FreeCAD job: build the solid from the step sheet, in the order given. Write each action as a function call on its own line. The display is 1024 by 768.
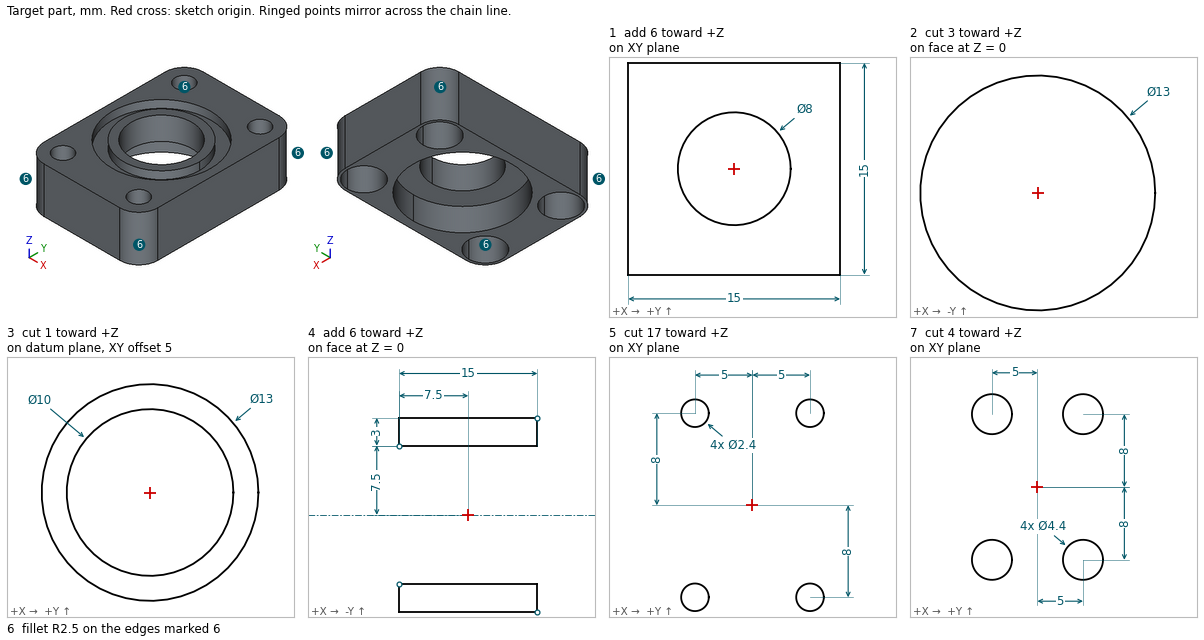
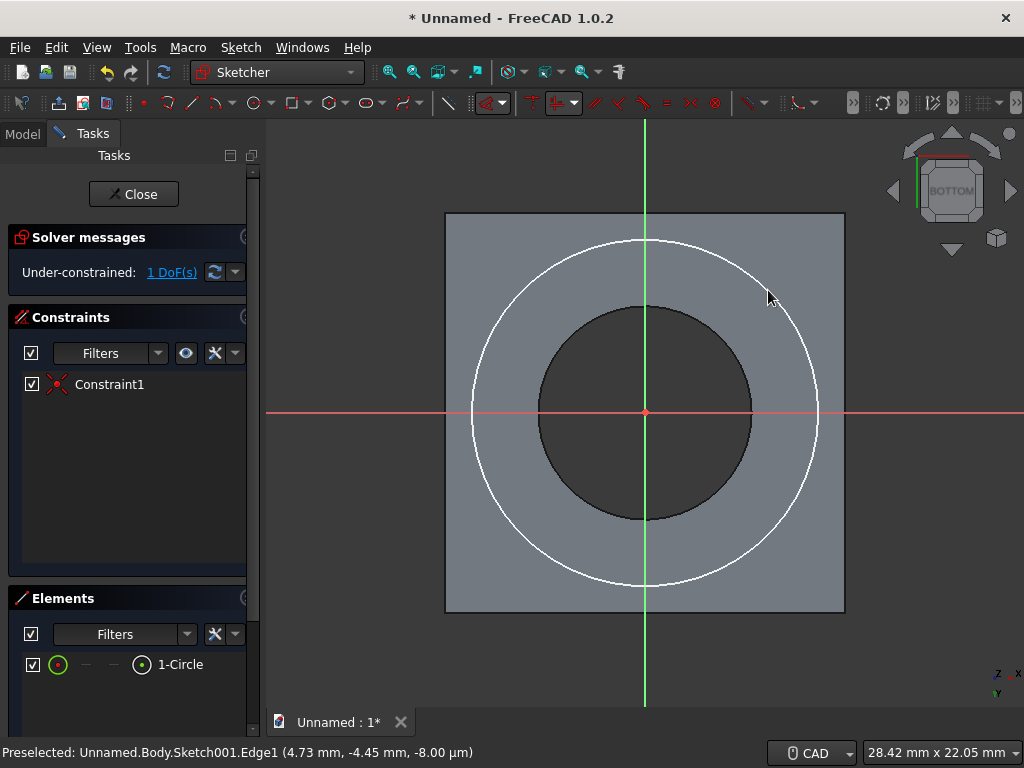
click(486, 104)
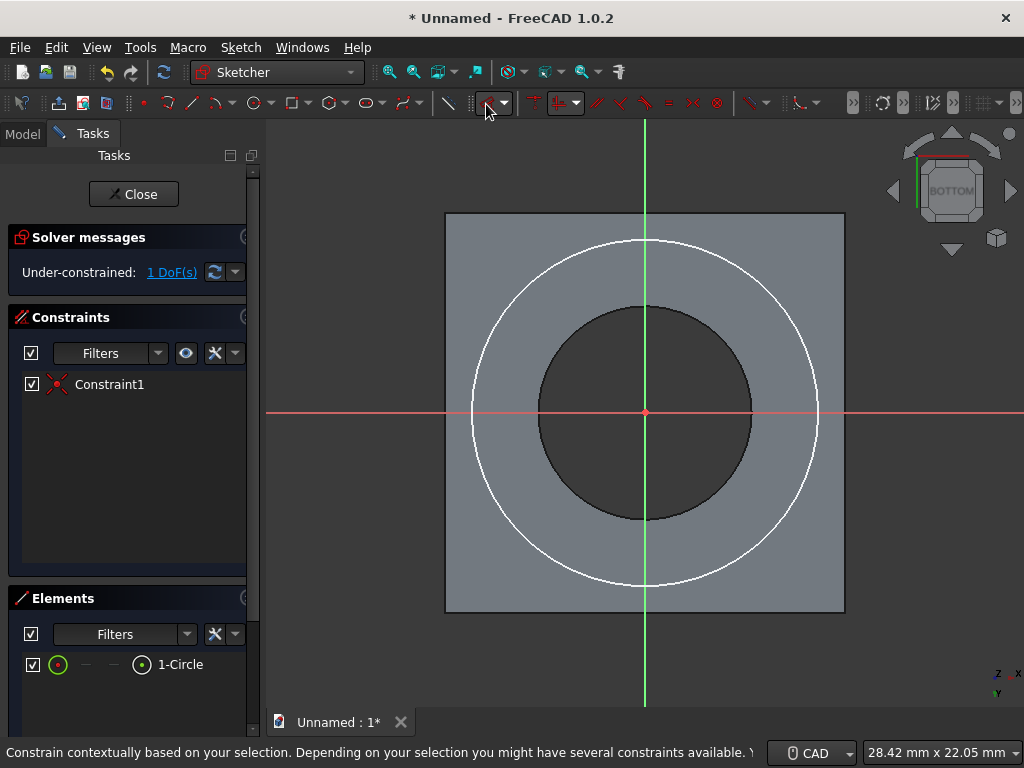
click(767, 290)
click(790, 267)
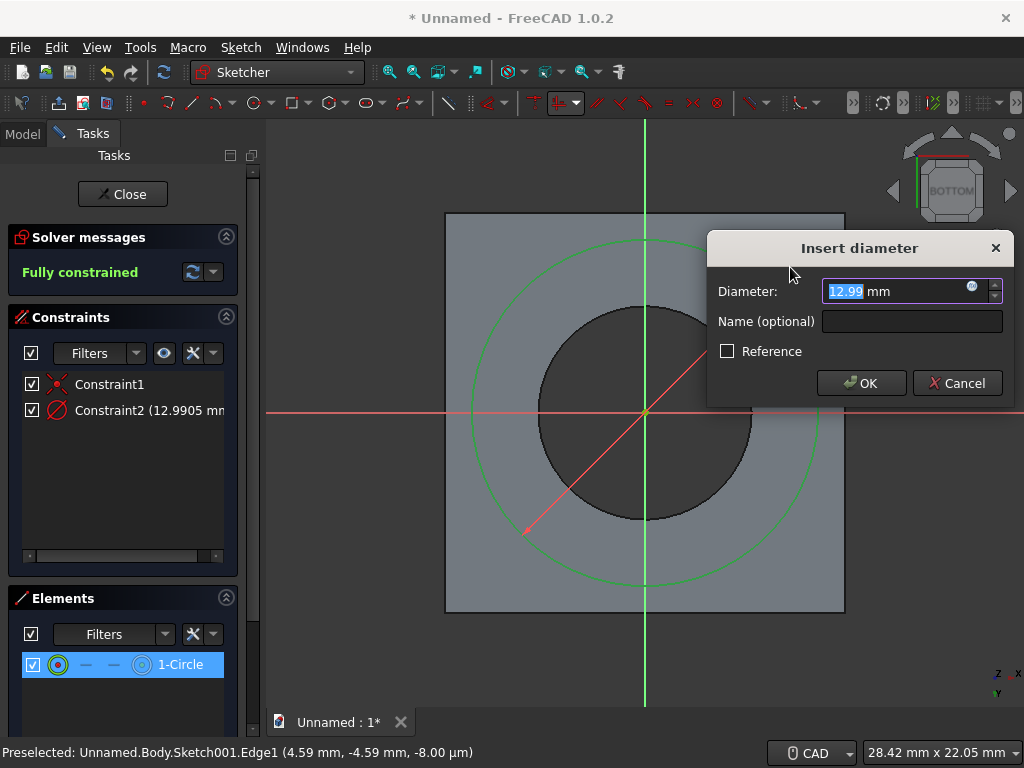
text(13)
key(Return)
key(Escape)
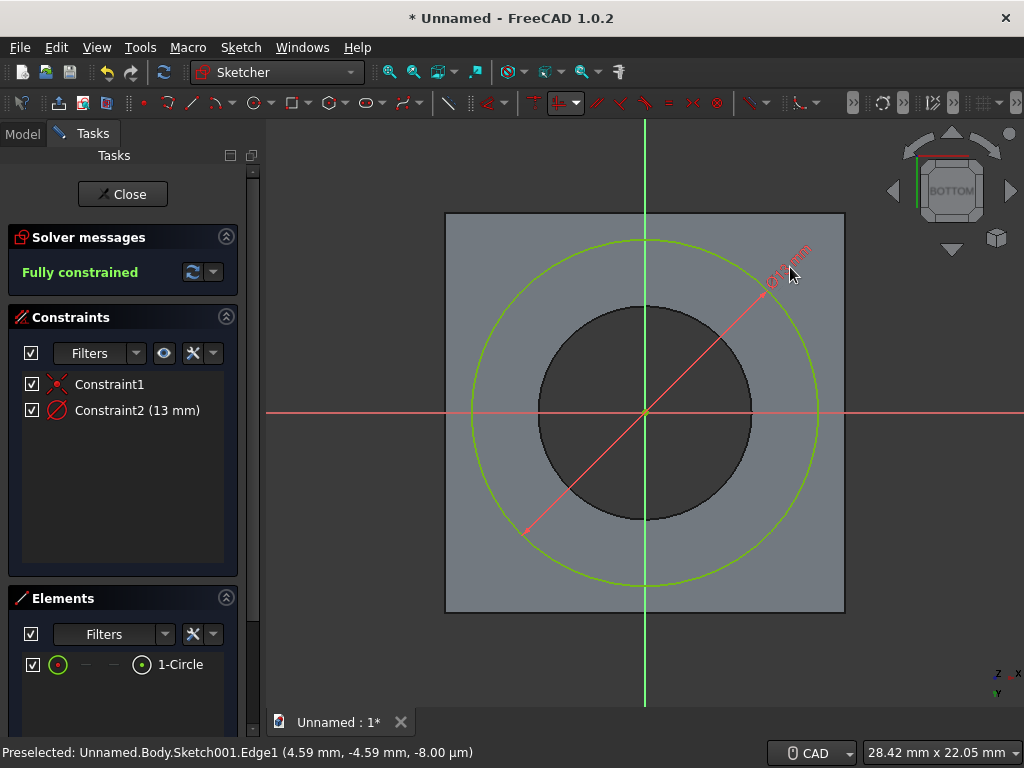
click(123, 194)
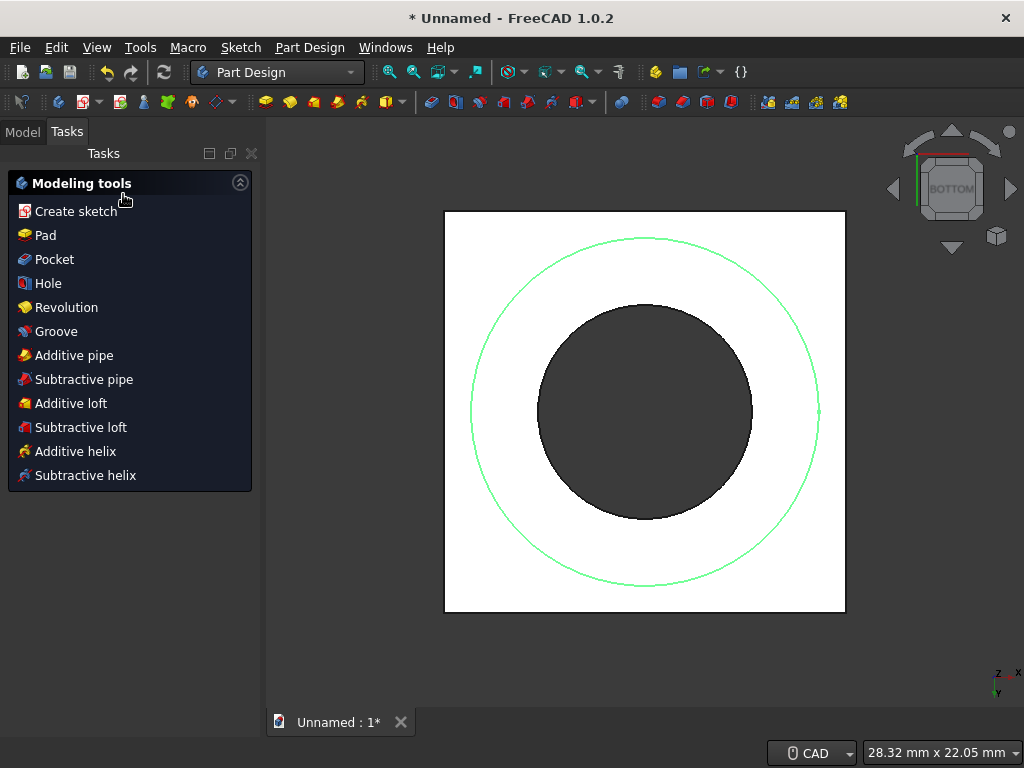
click(432, 102)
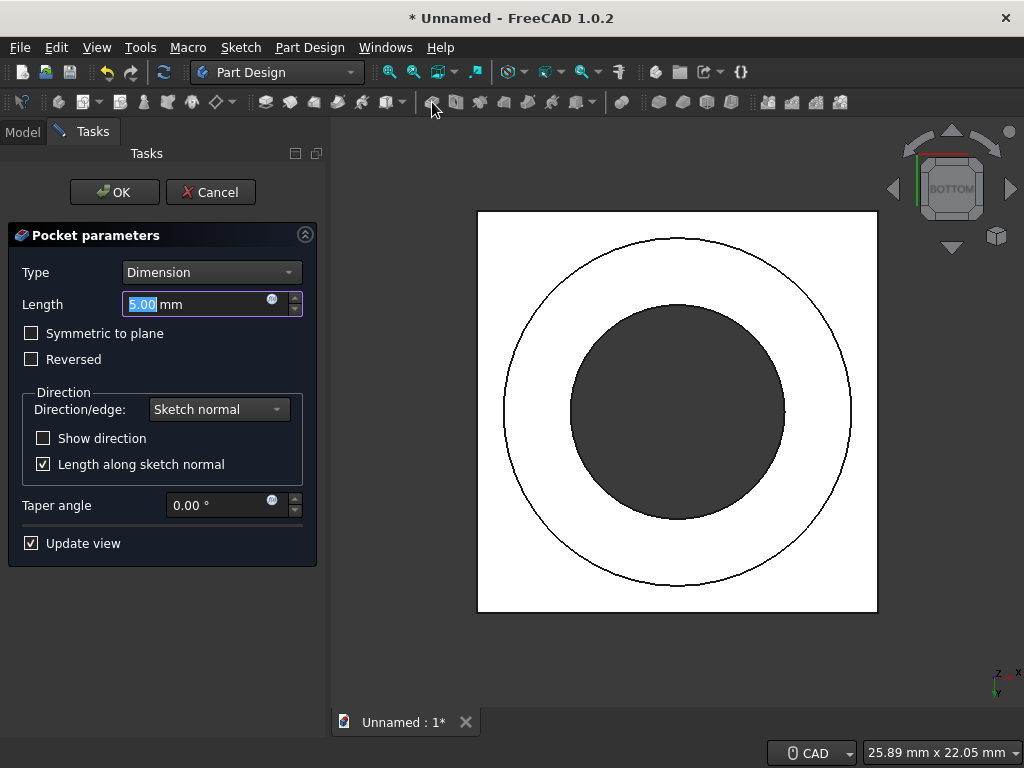
text(3)
key(Tab)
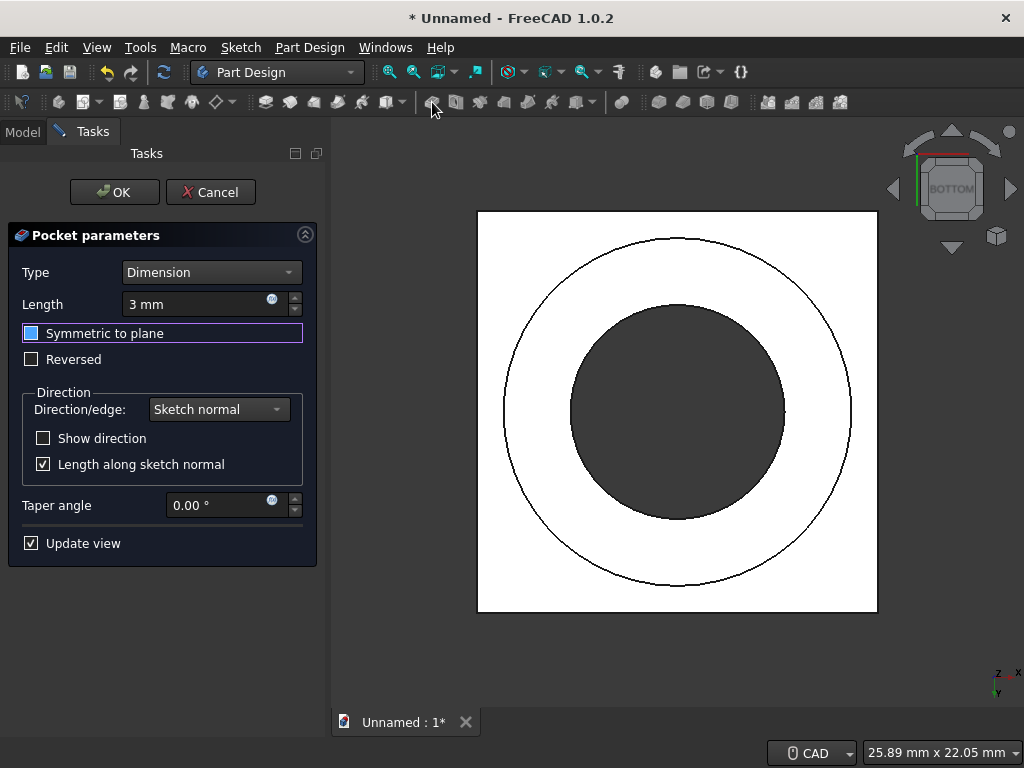
click(115, 192)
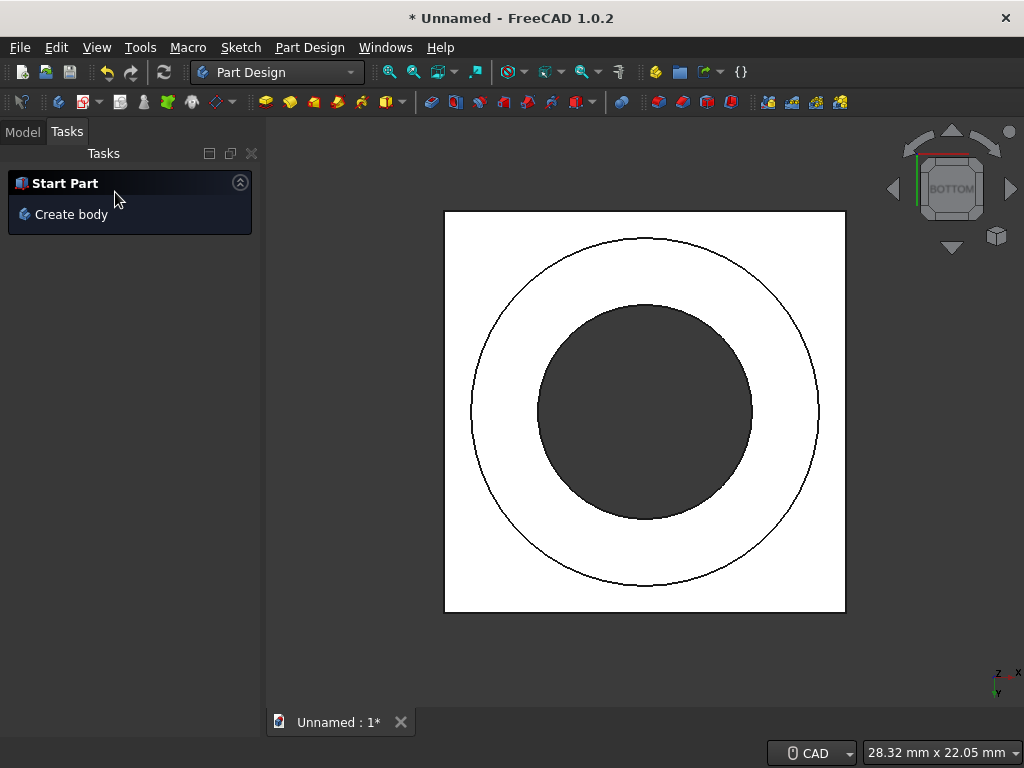
click(23, 131)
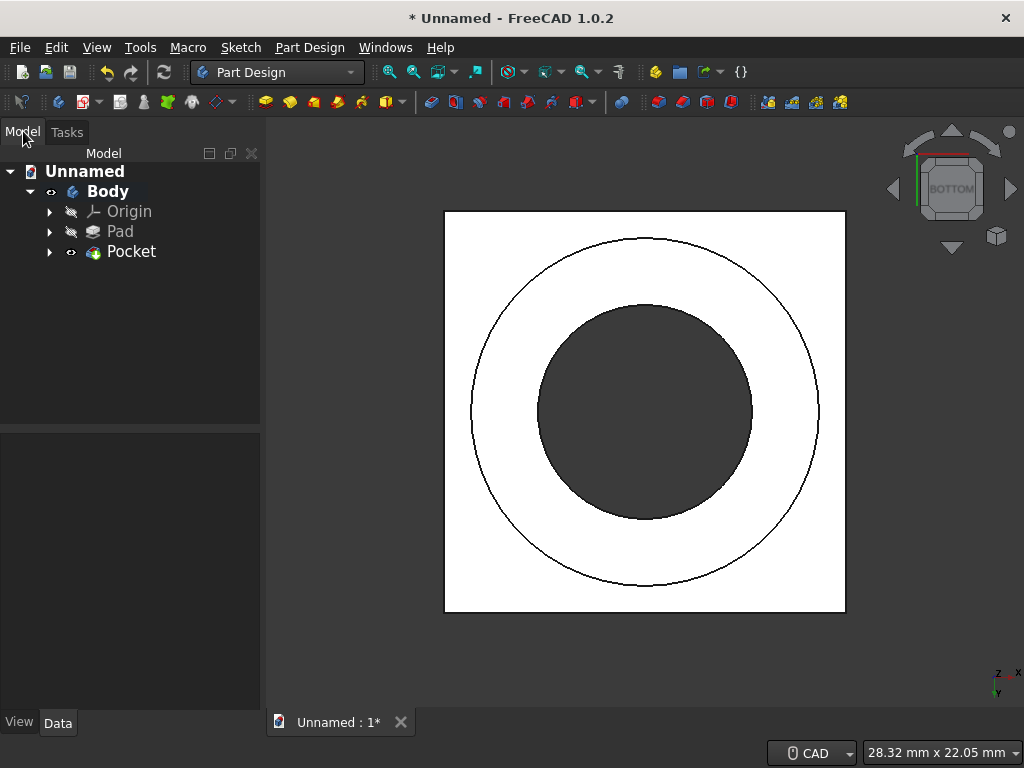
click(50, 212)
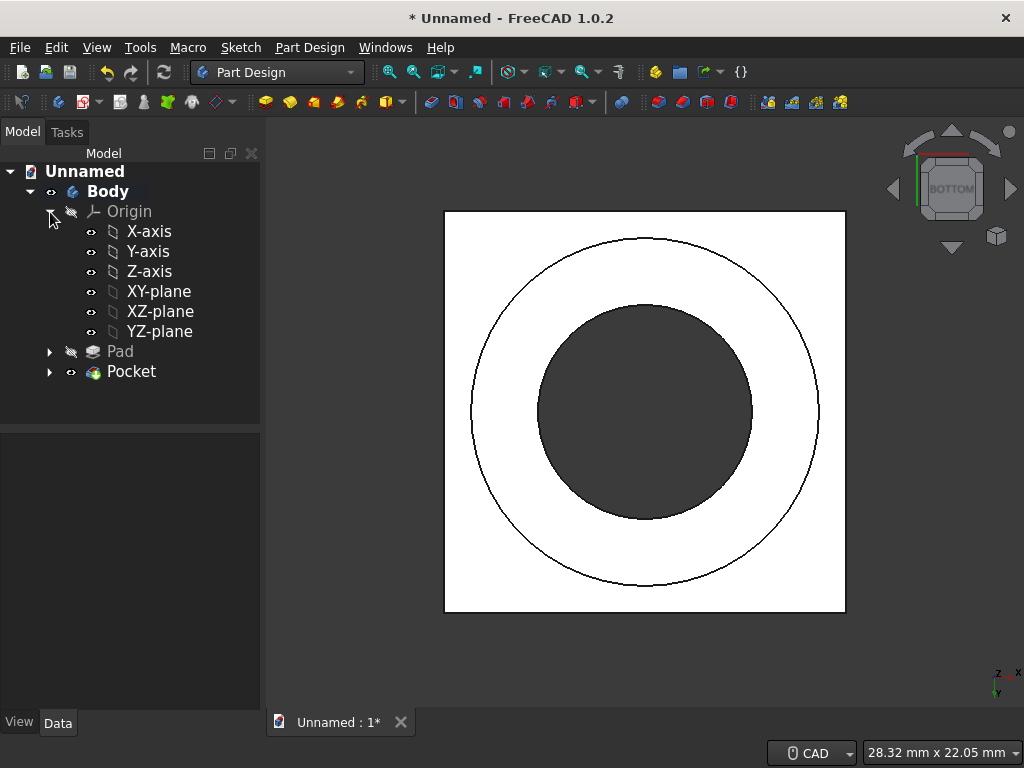
click(136, 292)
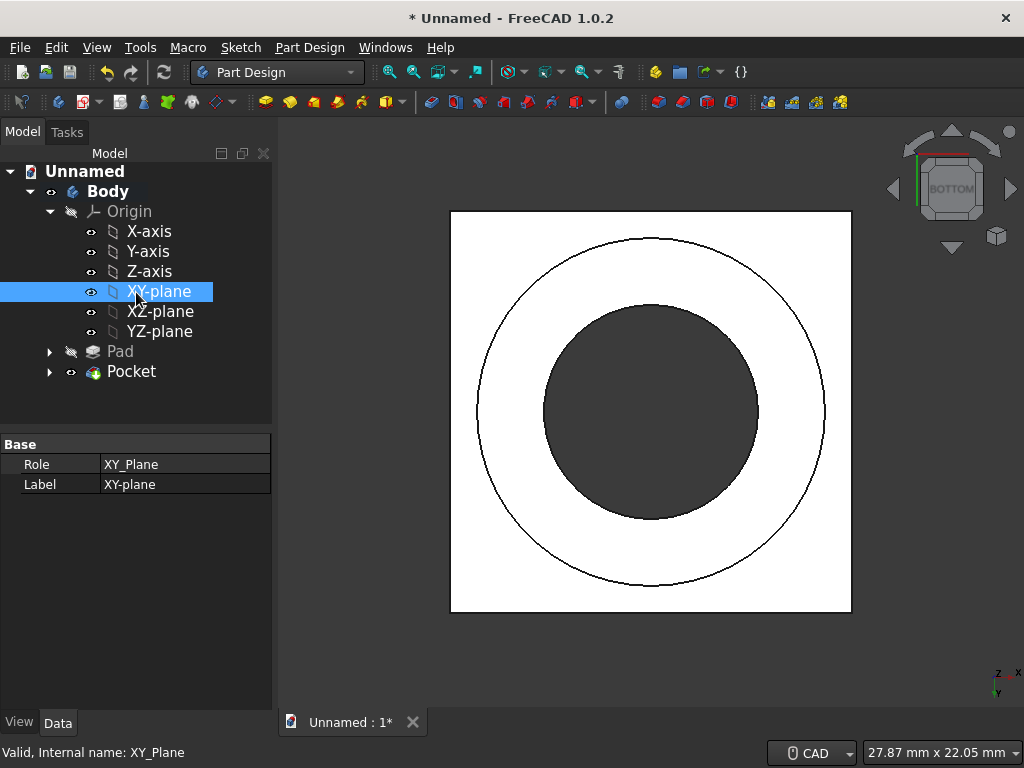
click(216, 102)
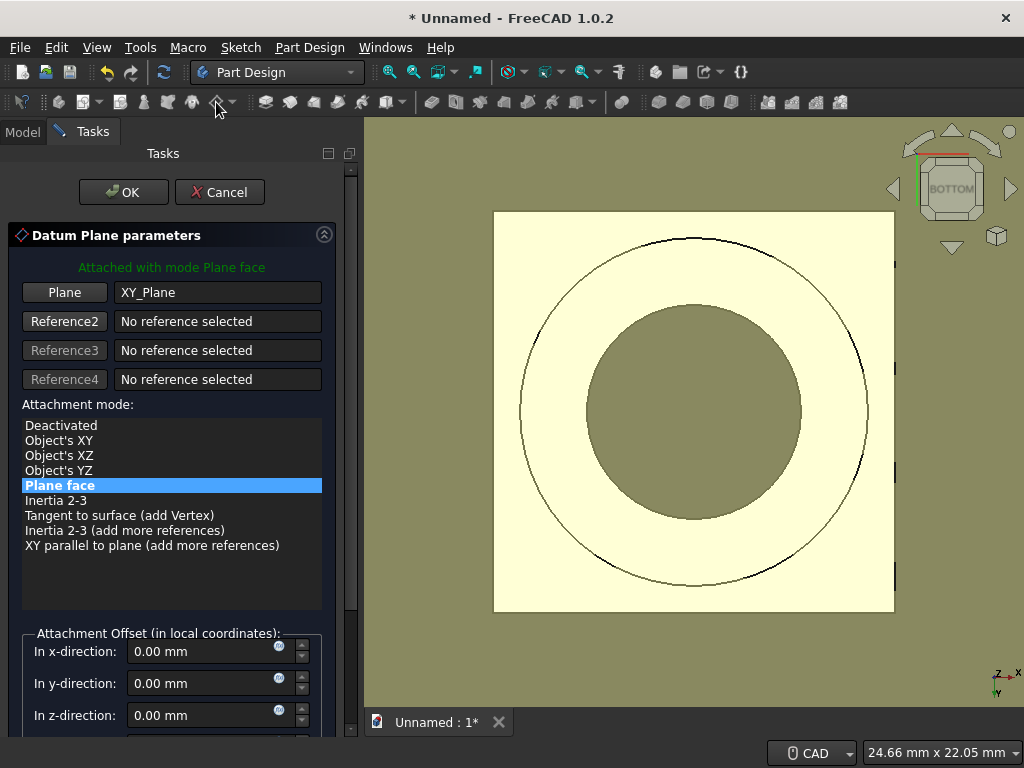
triple_click(210, 715)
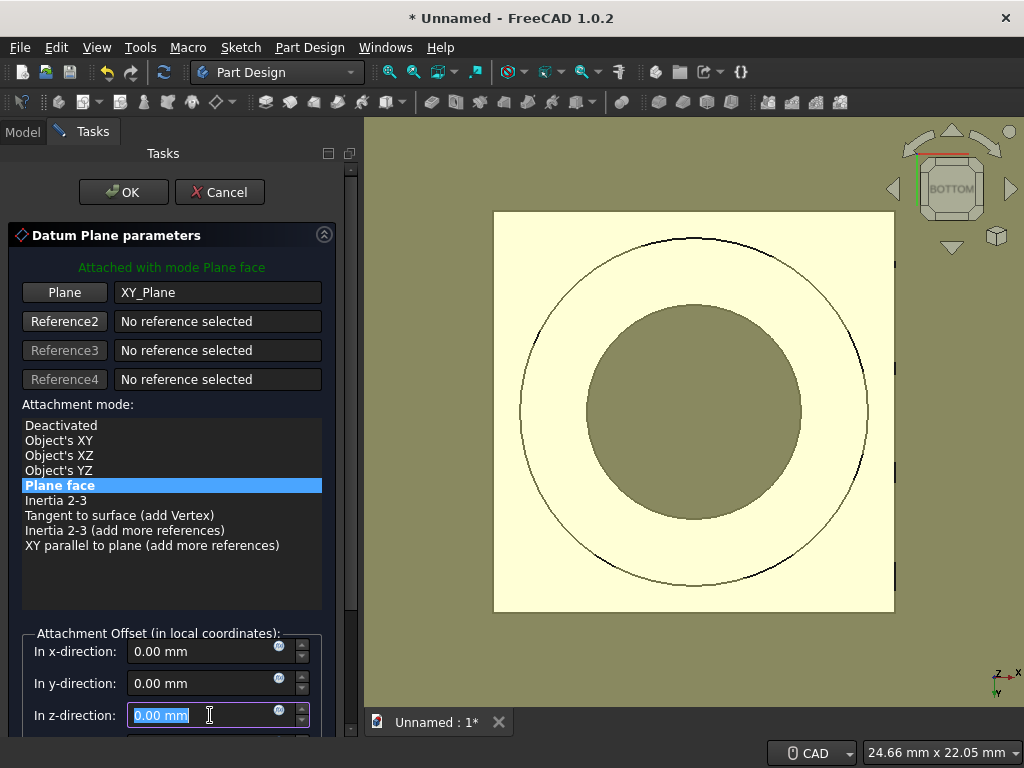
text(5)
key(Tab)